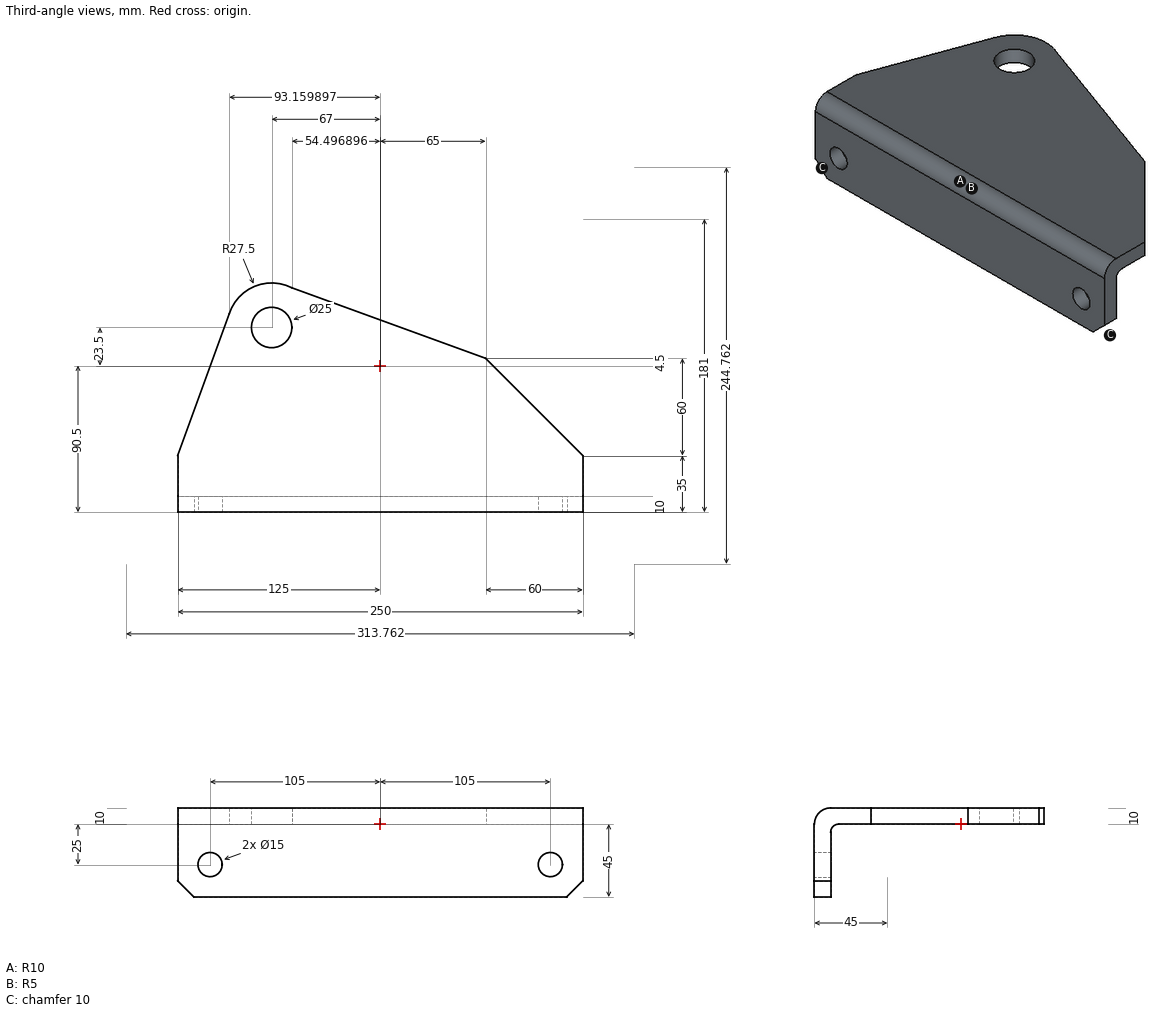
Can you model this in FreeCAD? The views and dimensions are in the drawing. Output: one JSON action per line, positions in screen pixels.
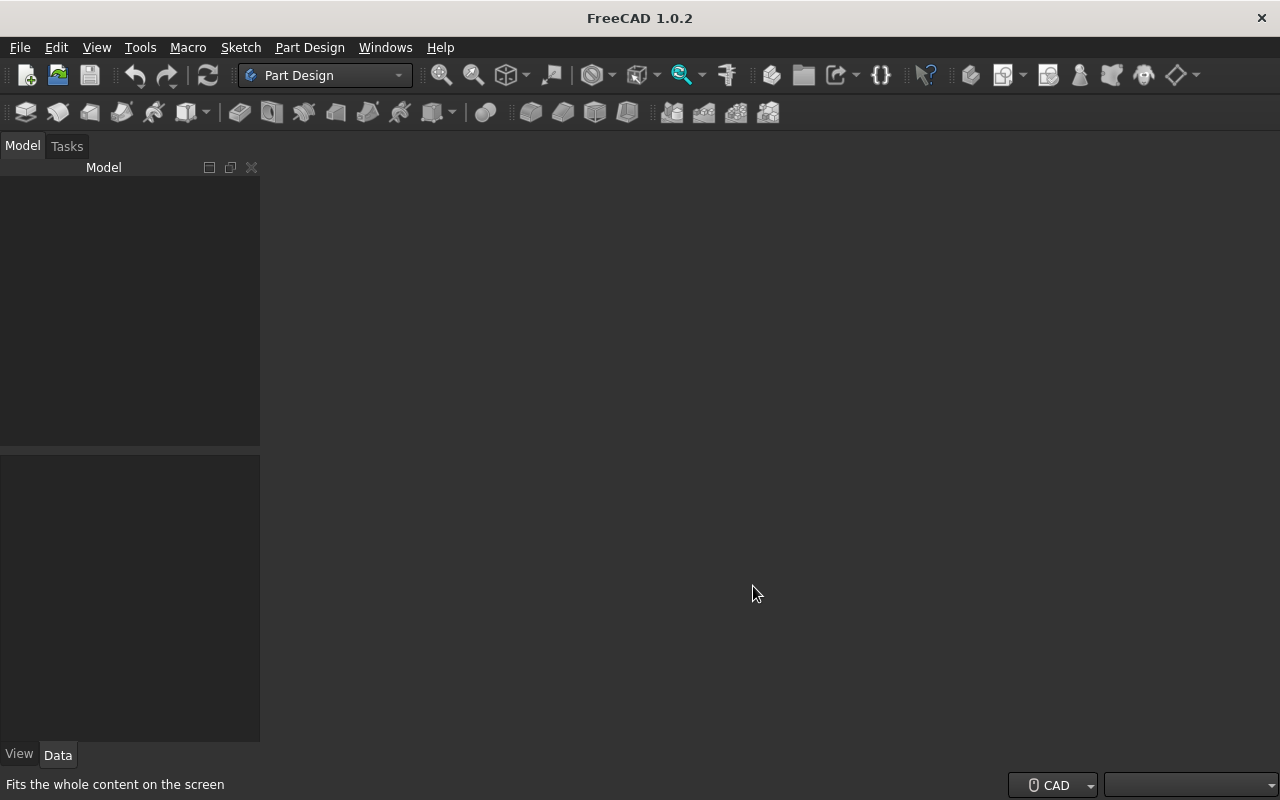
{"action": "key", "text": "ctrl+n"}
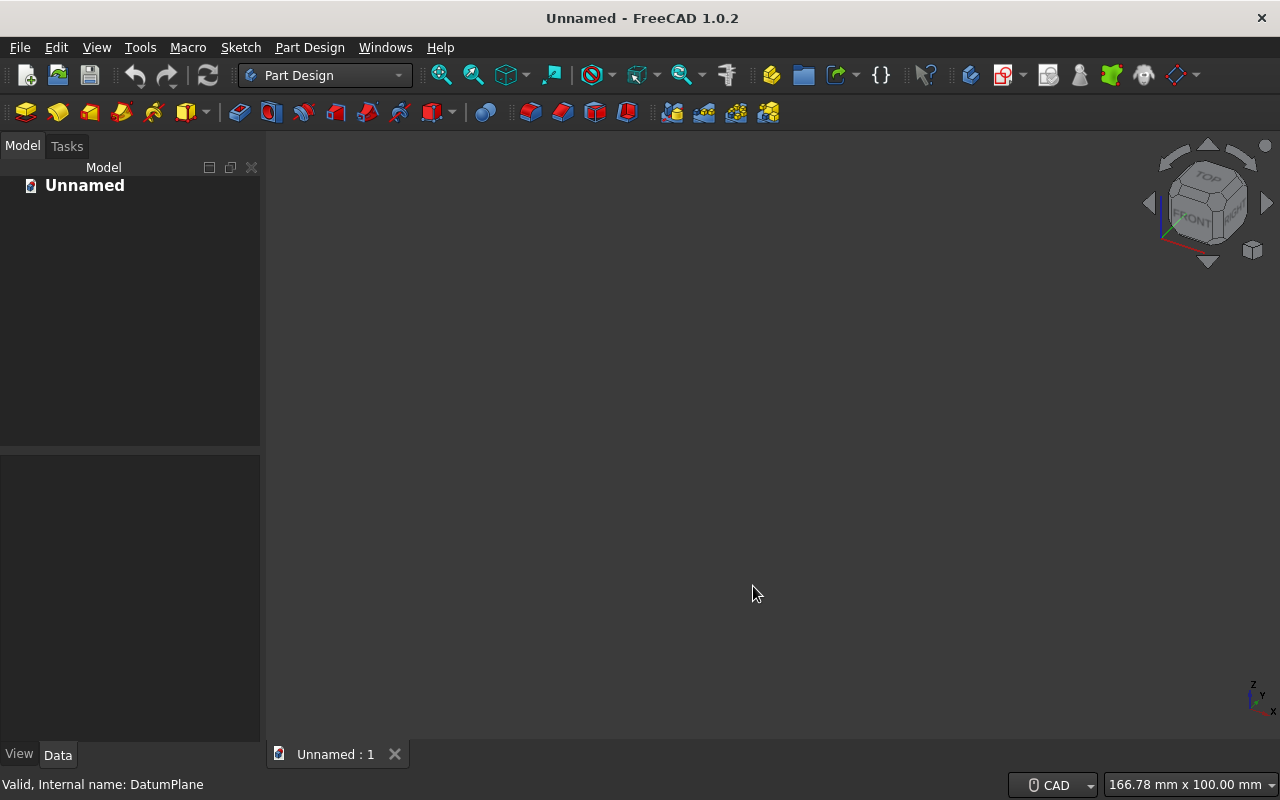
{"action": "left_click", "coordinate": [1004, 76]}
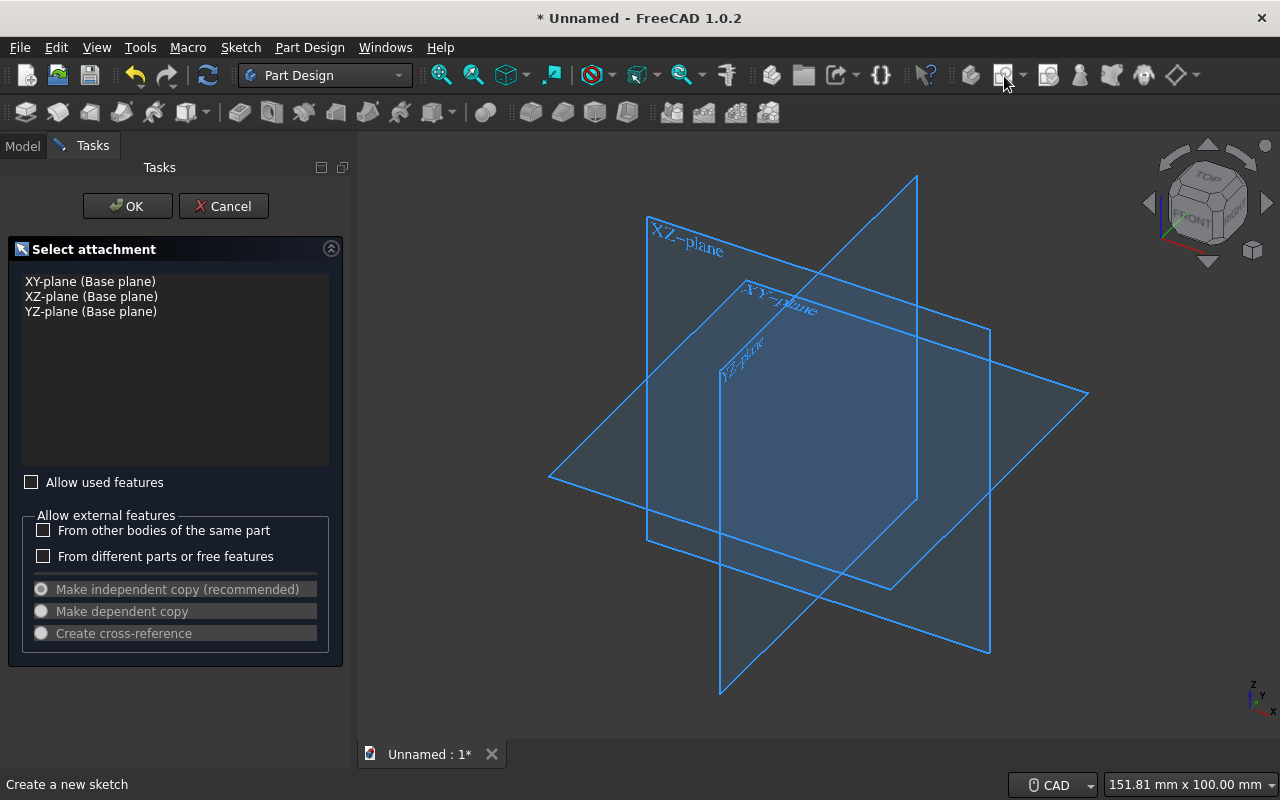
{"action": "left_click", "coordinate": [82, 282]}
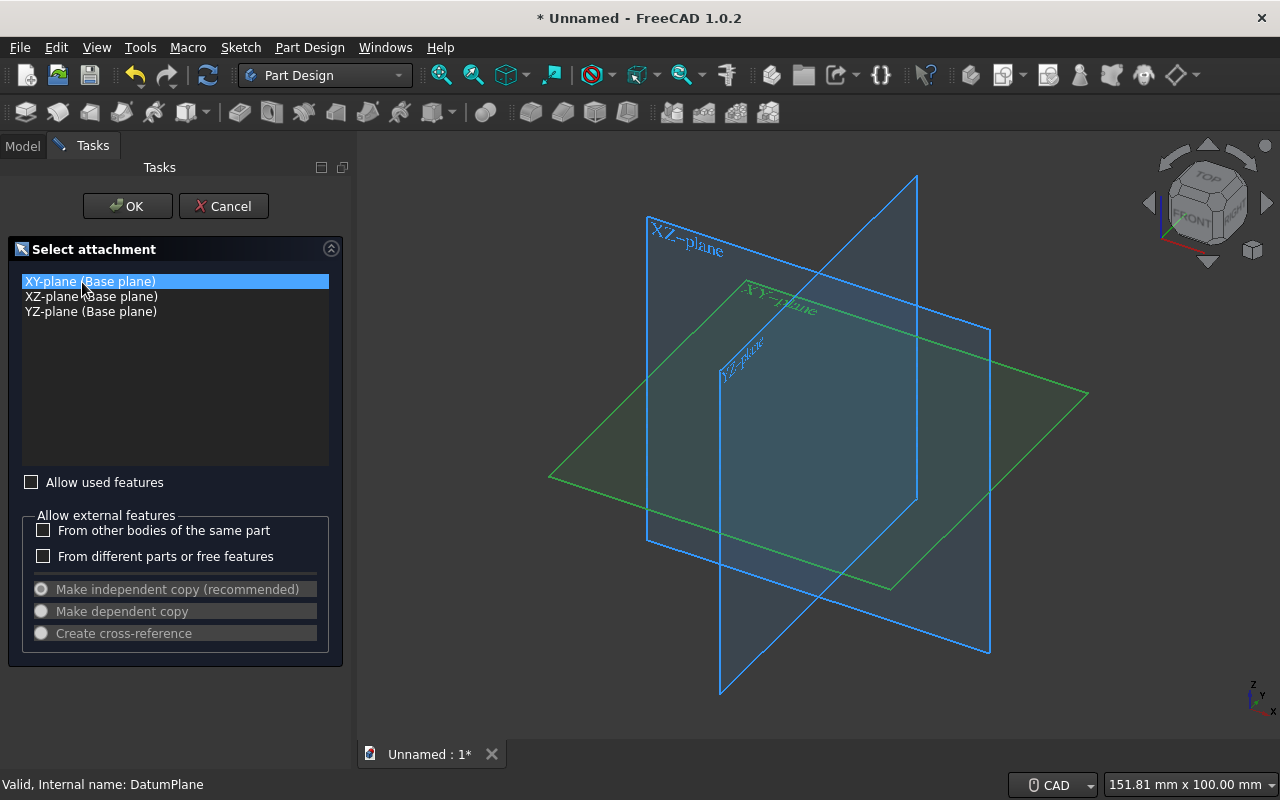
{"action": "left_click", "coordinate": [128, 206]}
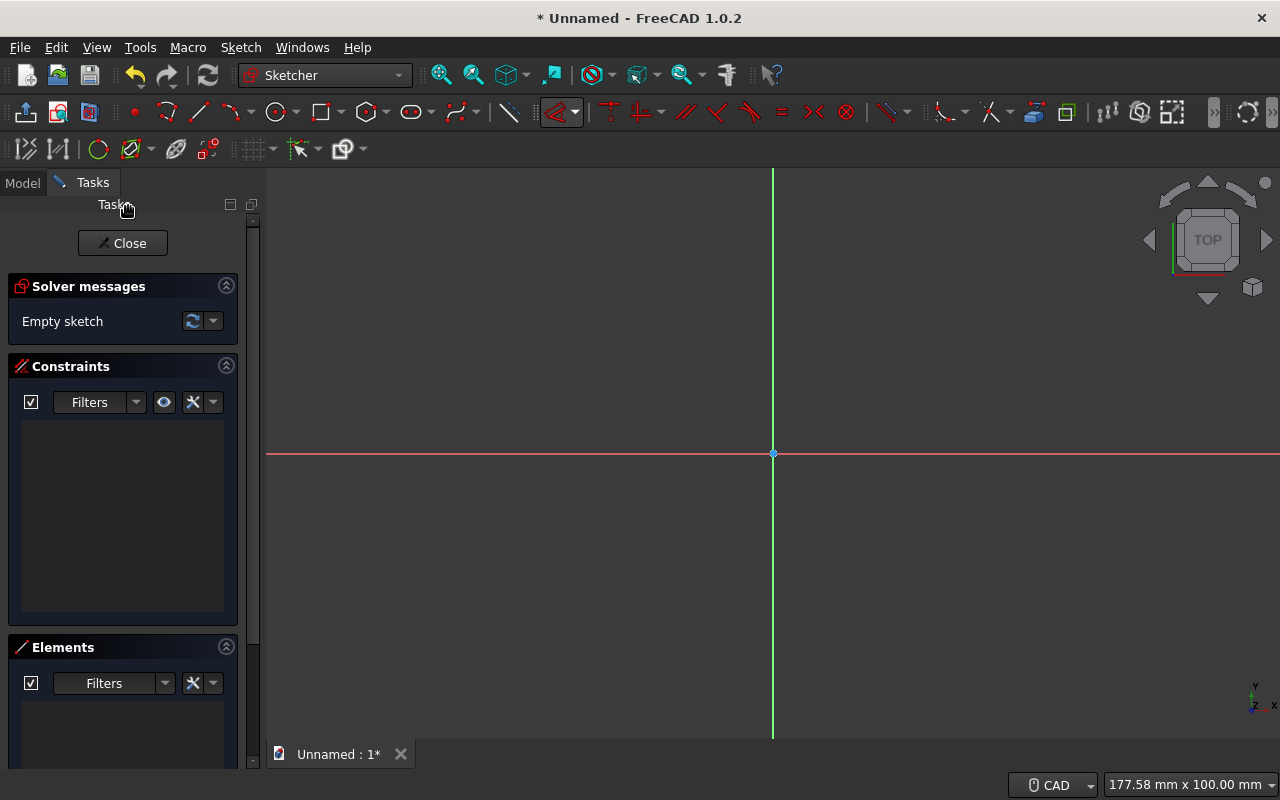
{"action": "scroll", "coordinate": [665, 453], "scroll_direction": "down", "scroll_amount": 5}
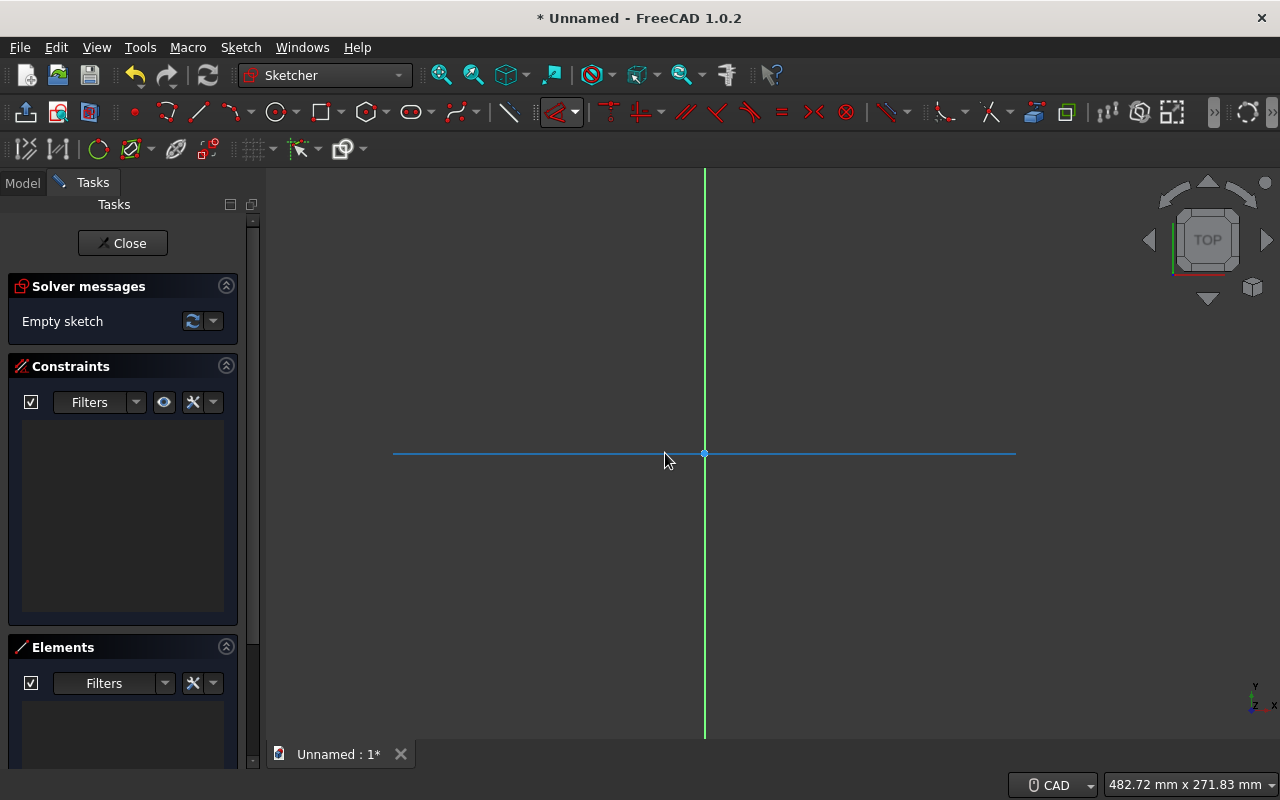
{"action": "left_click", "coordinate": [344, 112]}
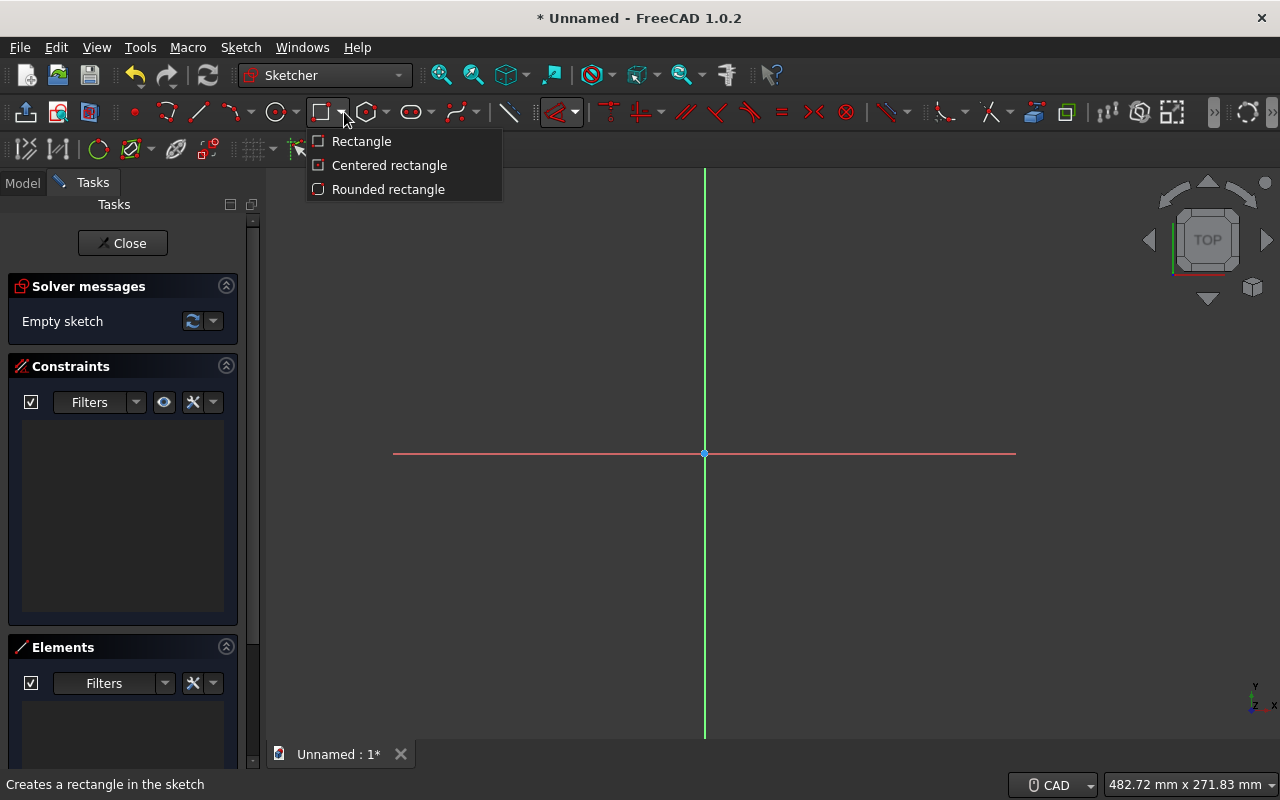
{"action": "left_click", "coordinate": [404, 165]}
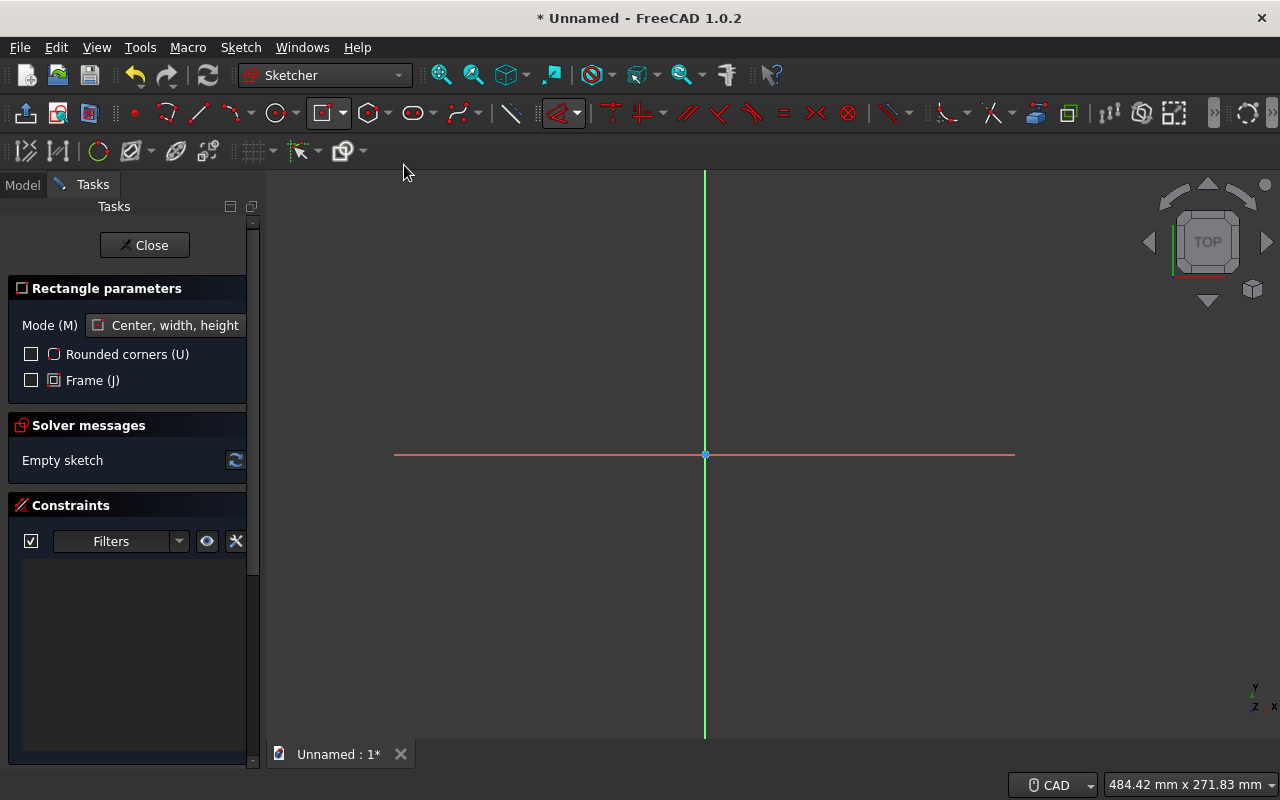
{"action": "left_click", "coordinate": [705, 454]}
{"action": "mouse_move", "coordinate": [967, 265]}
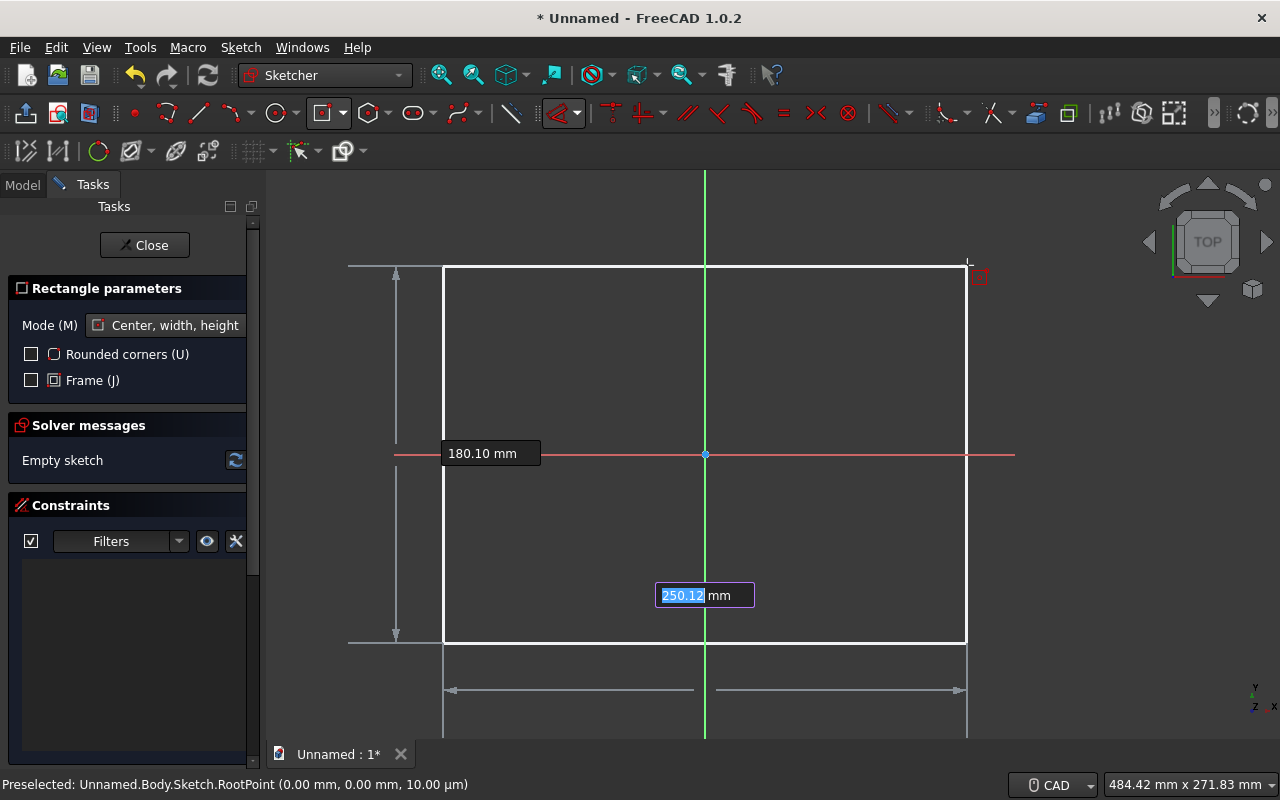
{"action": "type", "text": "250"}
{"action": "key", "text": "Tab"}
{"action": "type", "text": "181"}
{"action": "key", "text": "Return"}
{"action": "key", "text": "Escape"}